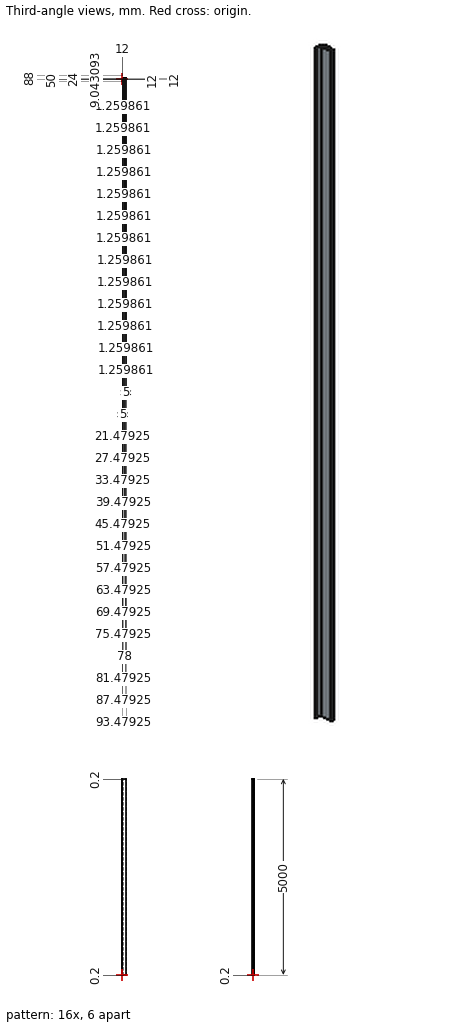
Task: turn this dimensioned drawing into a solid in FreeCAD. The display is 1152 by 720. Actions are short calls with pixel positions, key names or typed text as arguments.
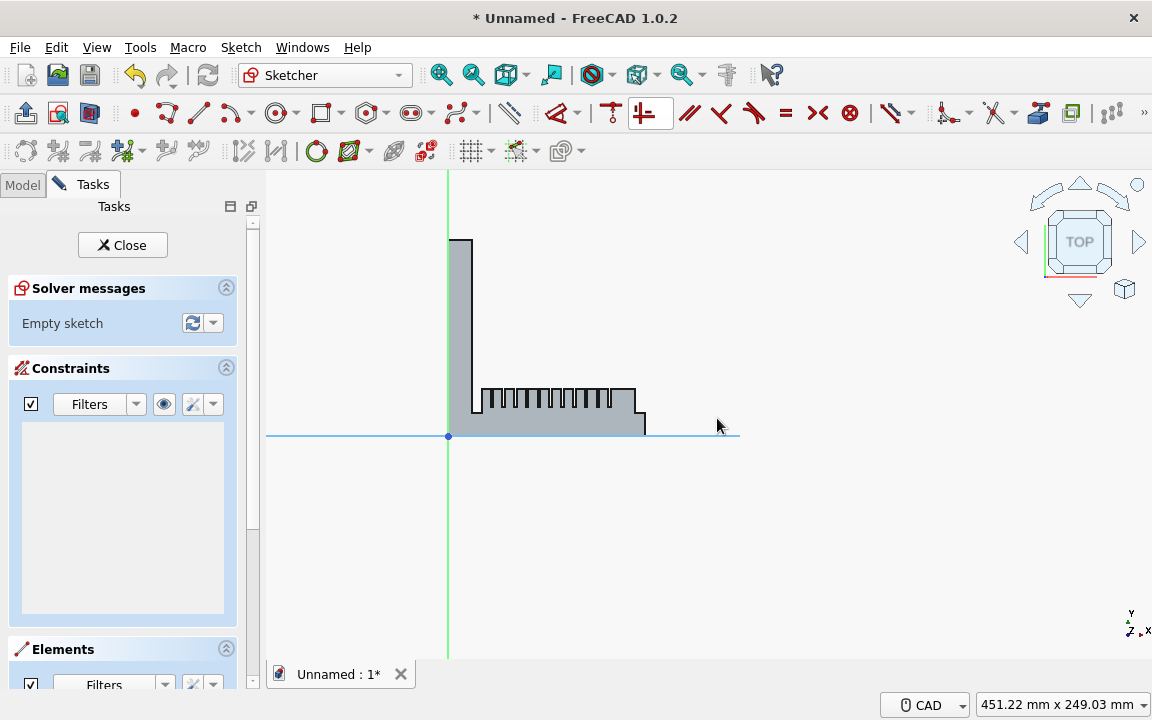
scroll(620, 397, up, 14)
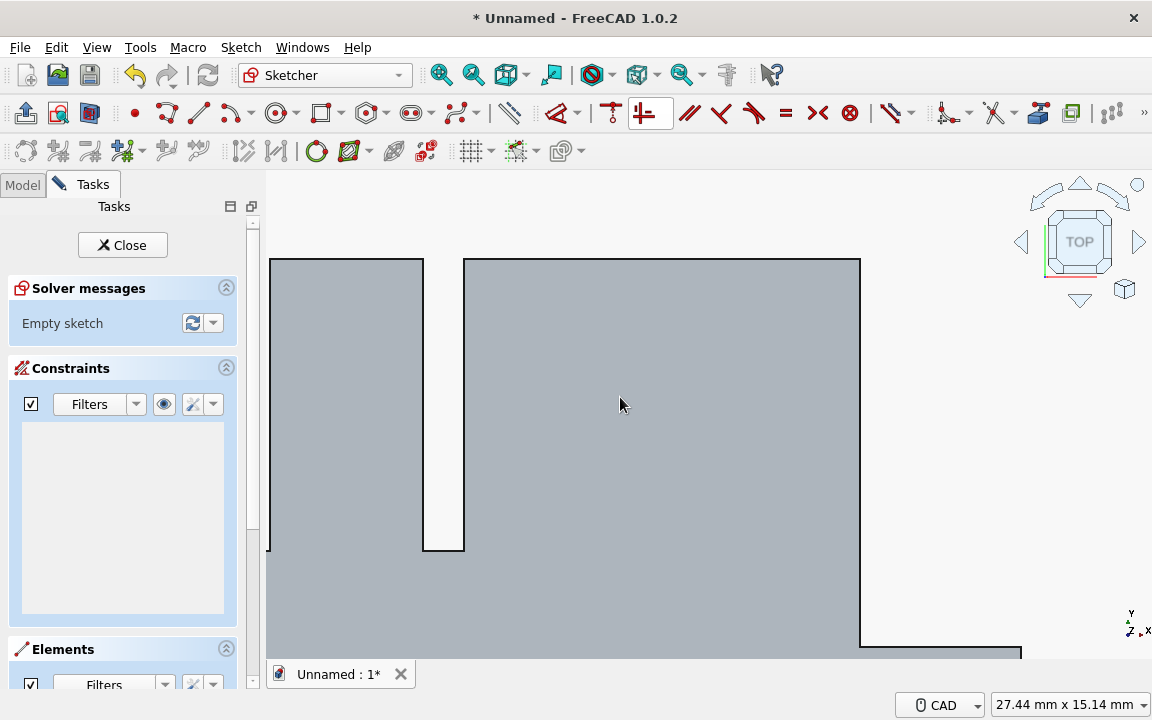
click(322, 114)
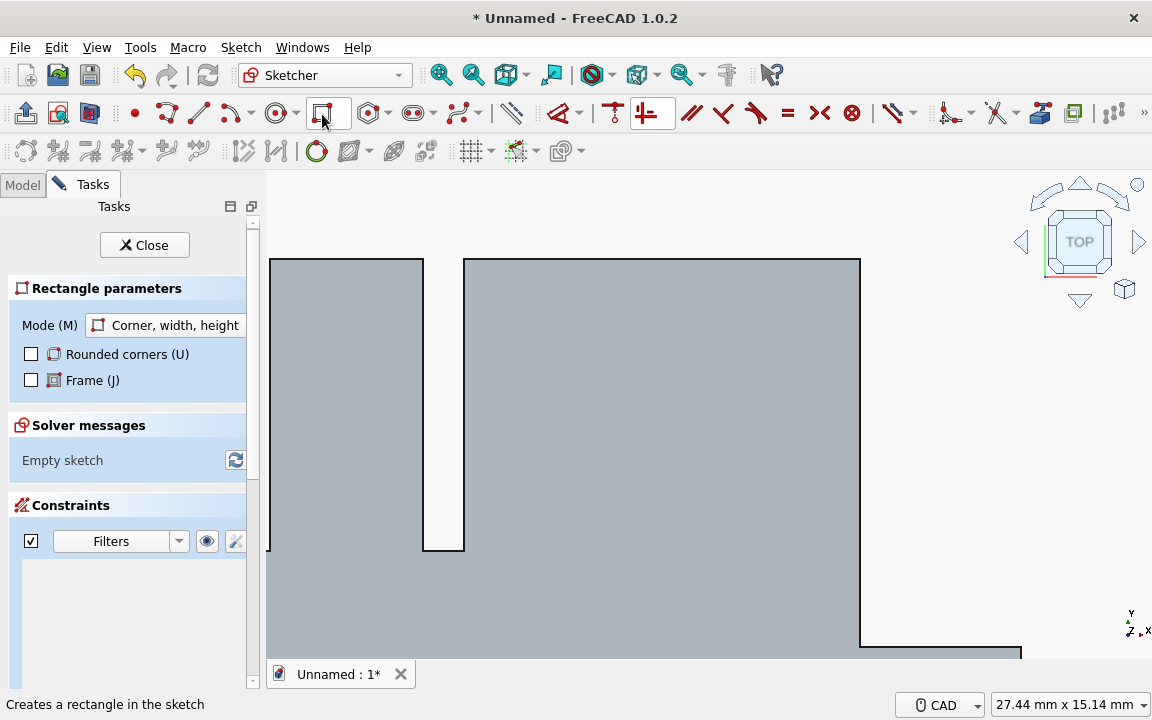
click(617, 259)
click(658, 551)
key(Escape)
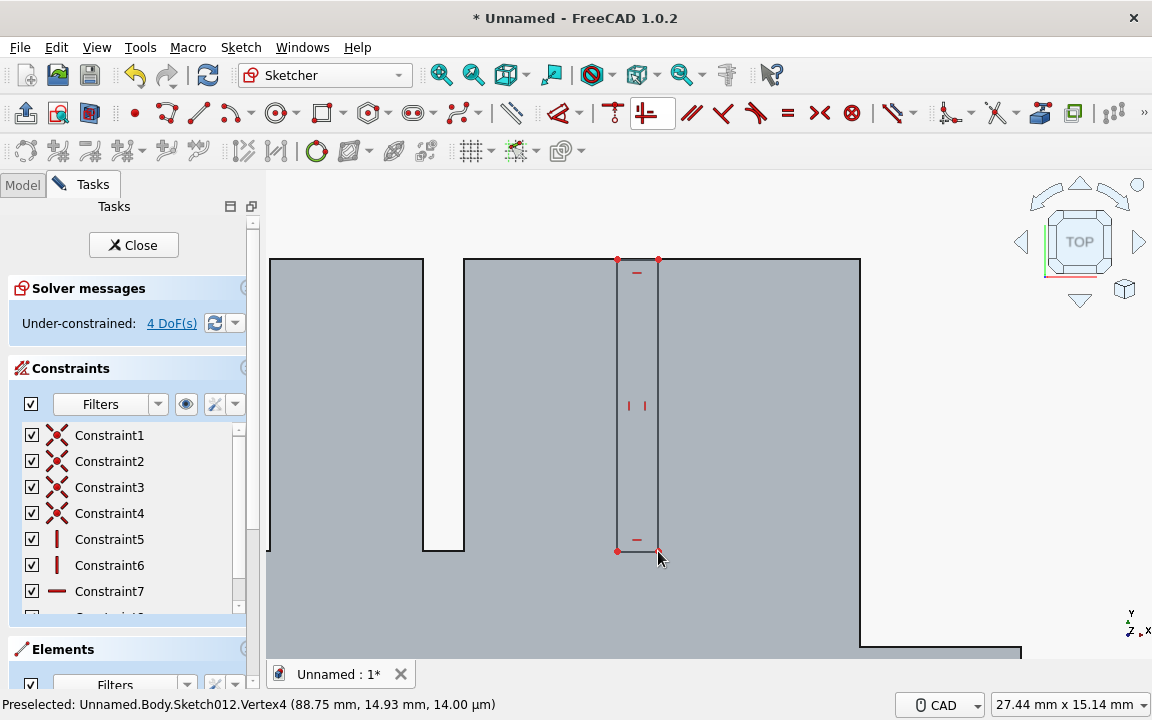
click(558, 114)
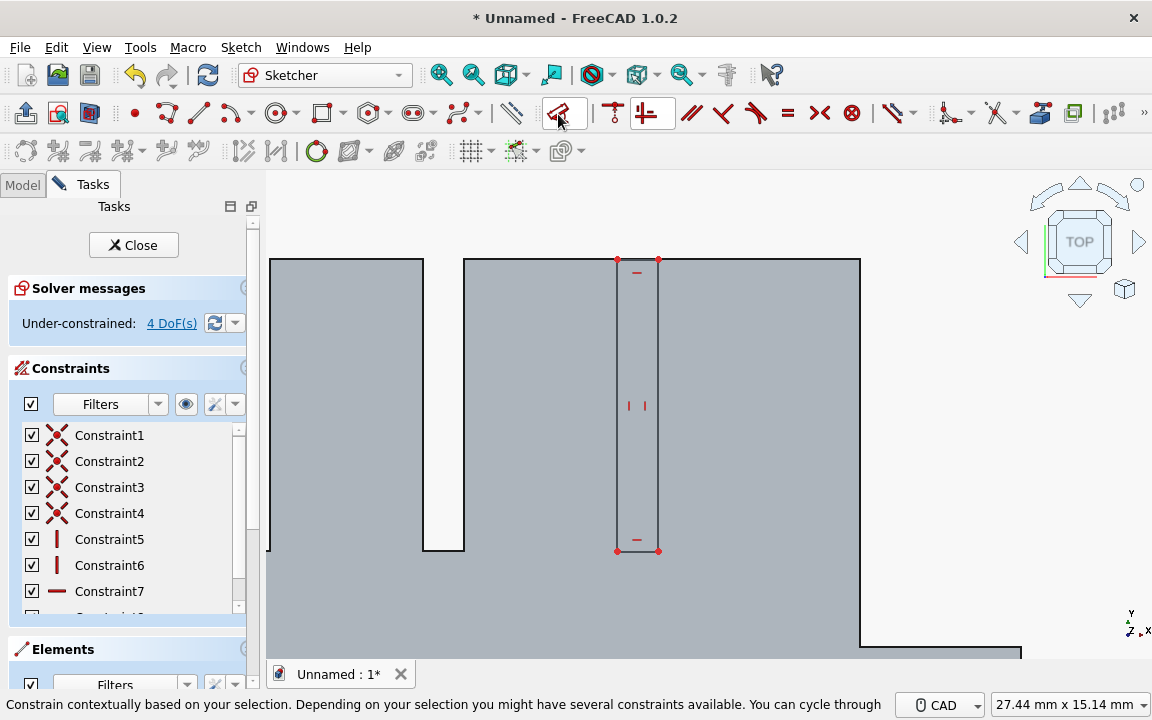
click(617, 260)
click(651, 575)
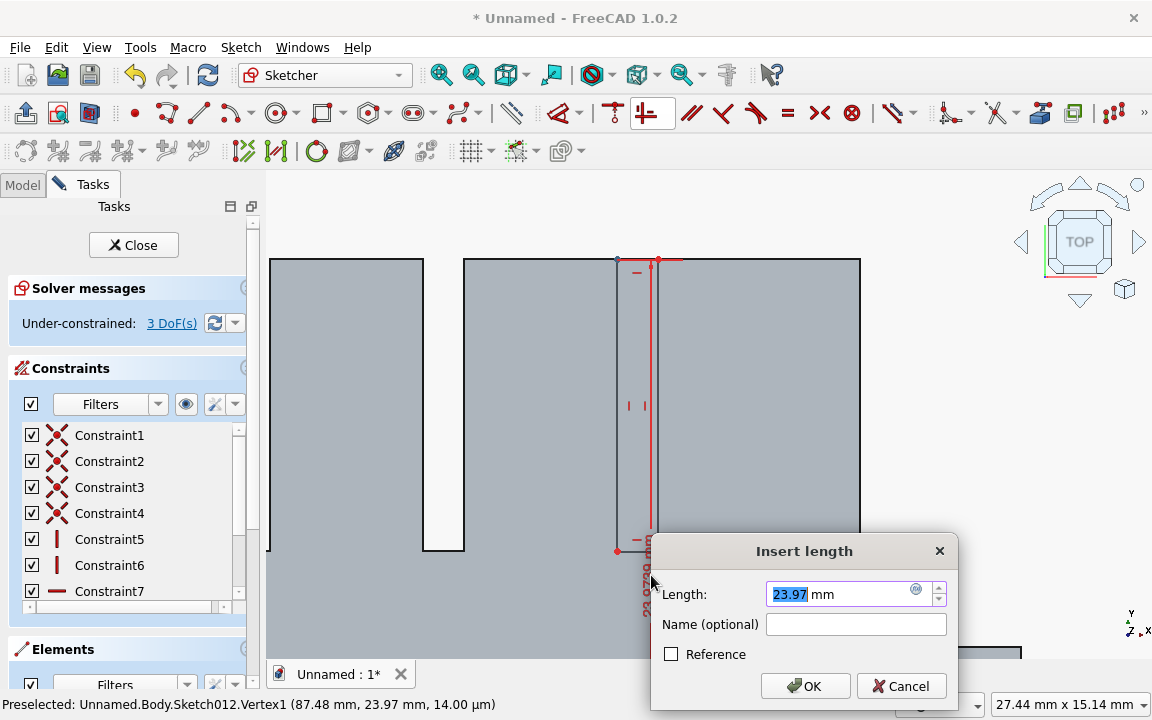
text(24)
key(Return)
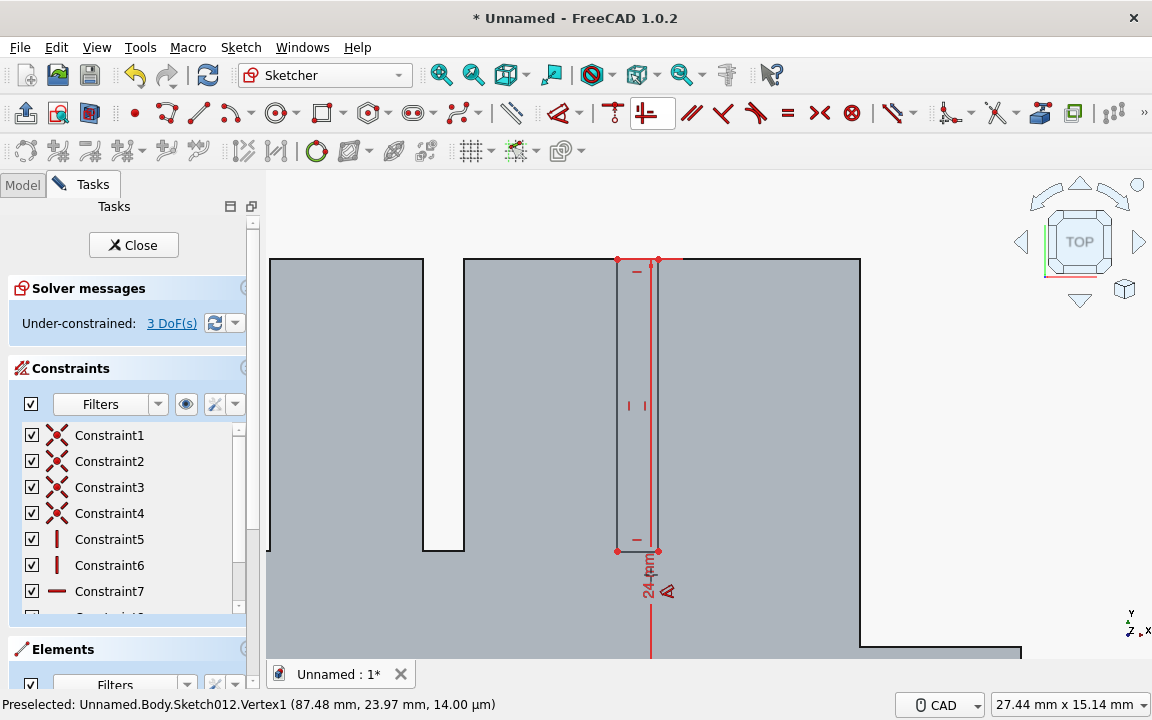
click(617, 347)
click(583, 406)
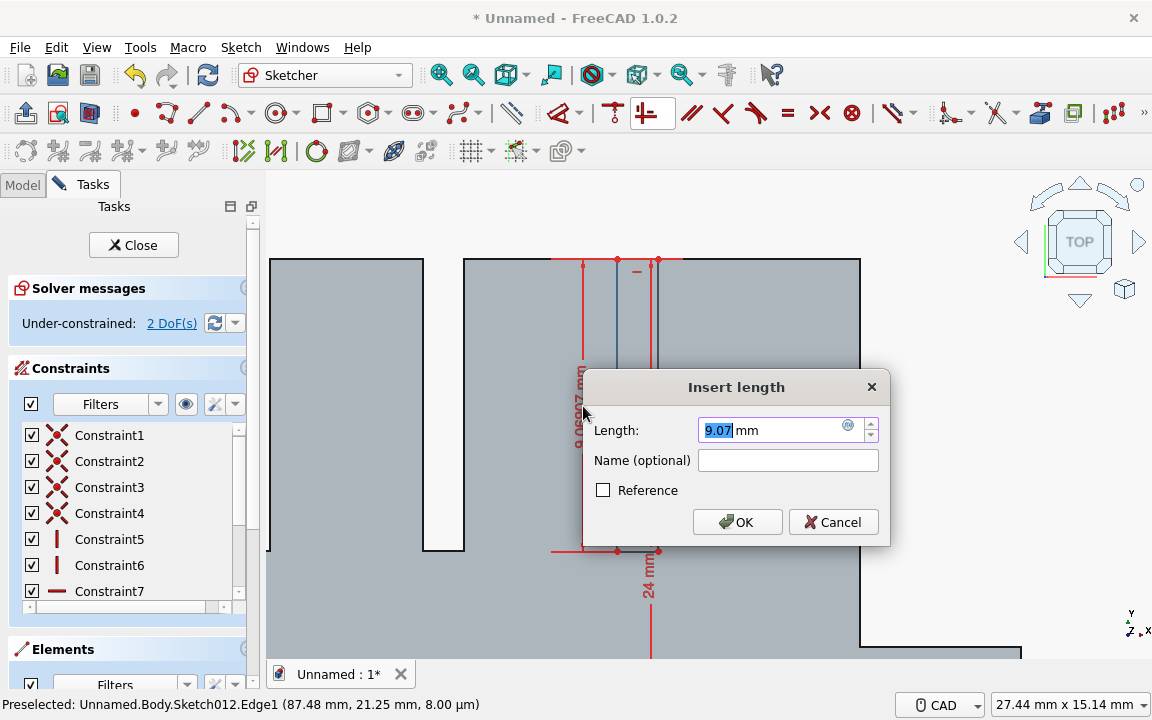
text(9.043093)
key(Return)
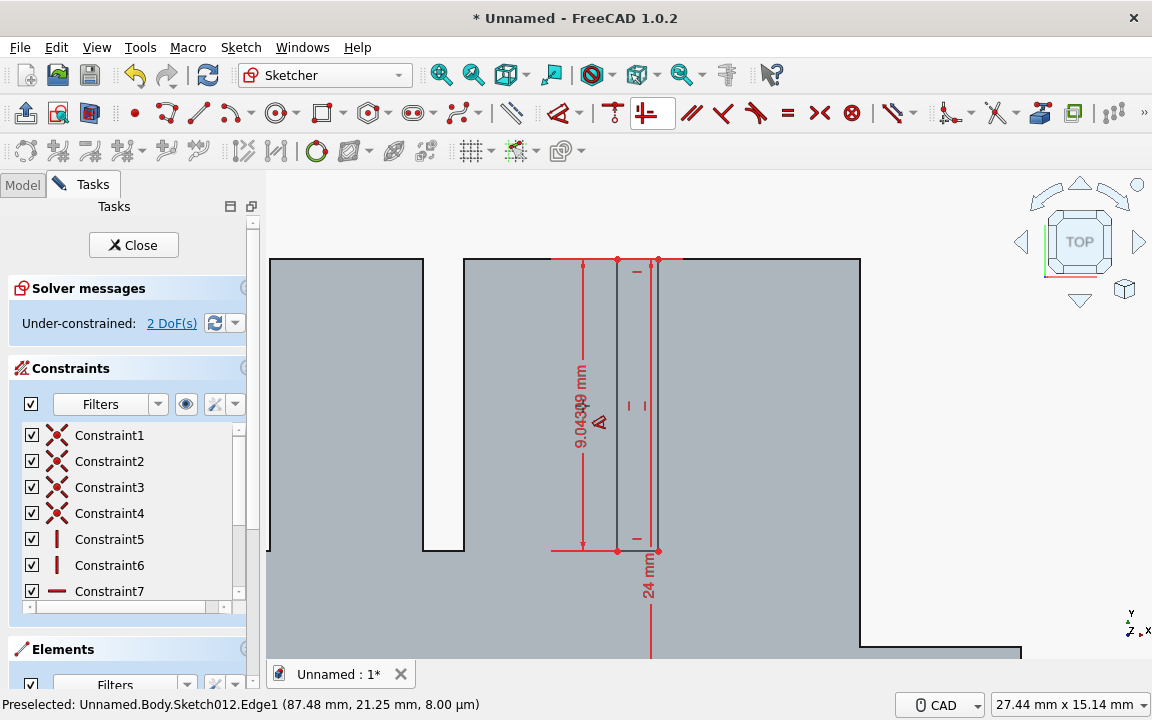
click(629, 551)
click(637, 517)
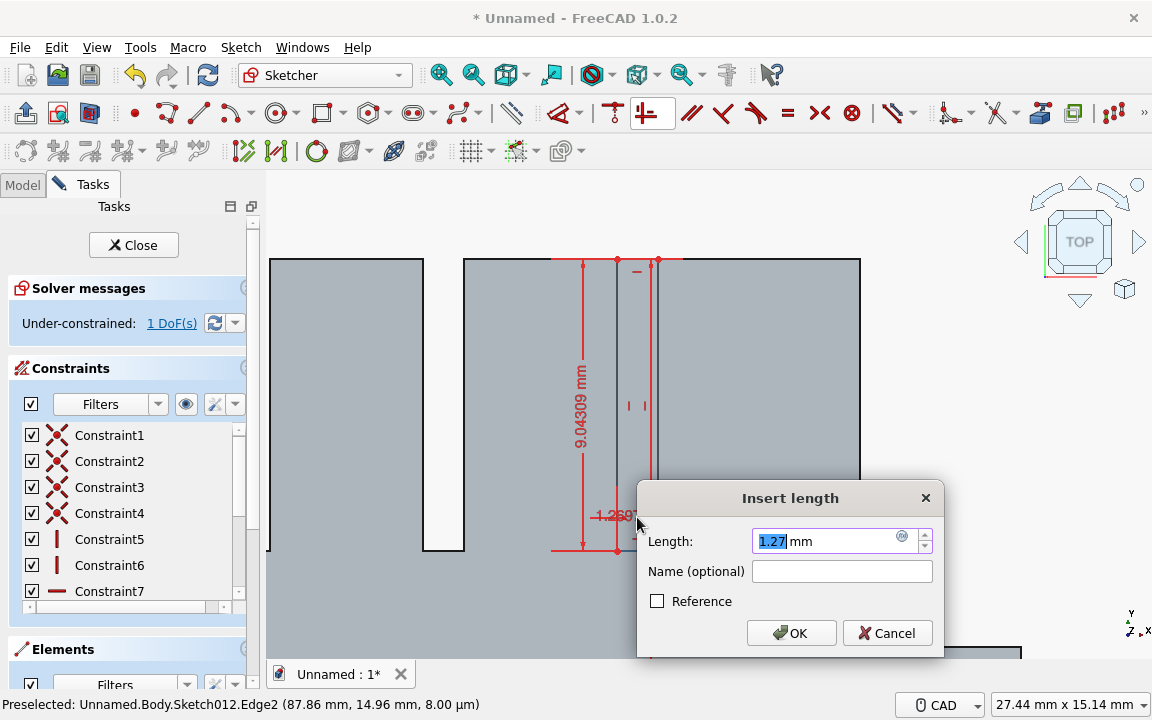
text(1.259861)
key(Return)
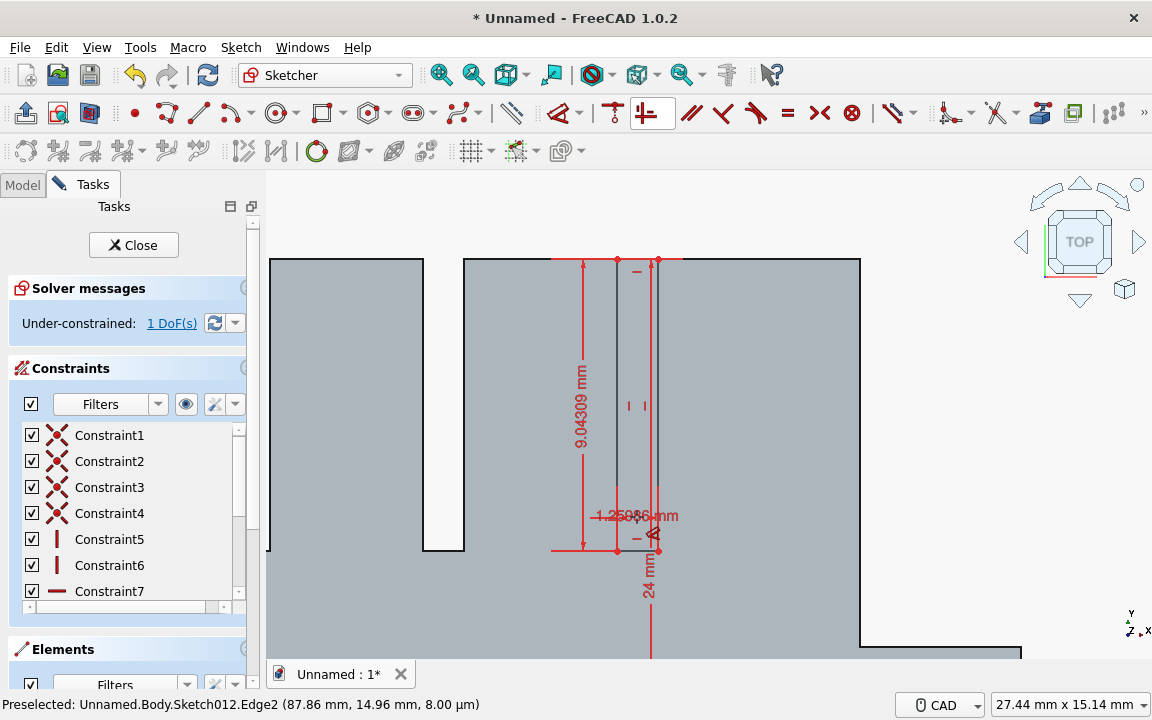
click(617, 259)
click(456, 225)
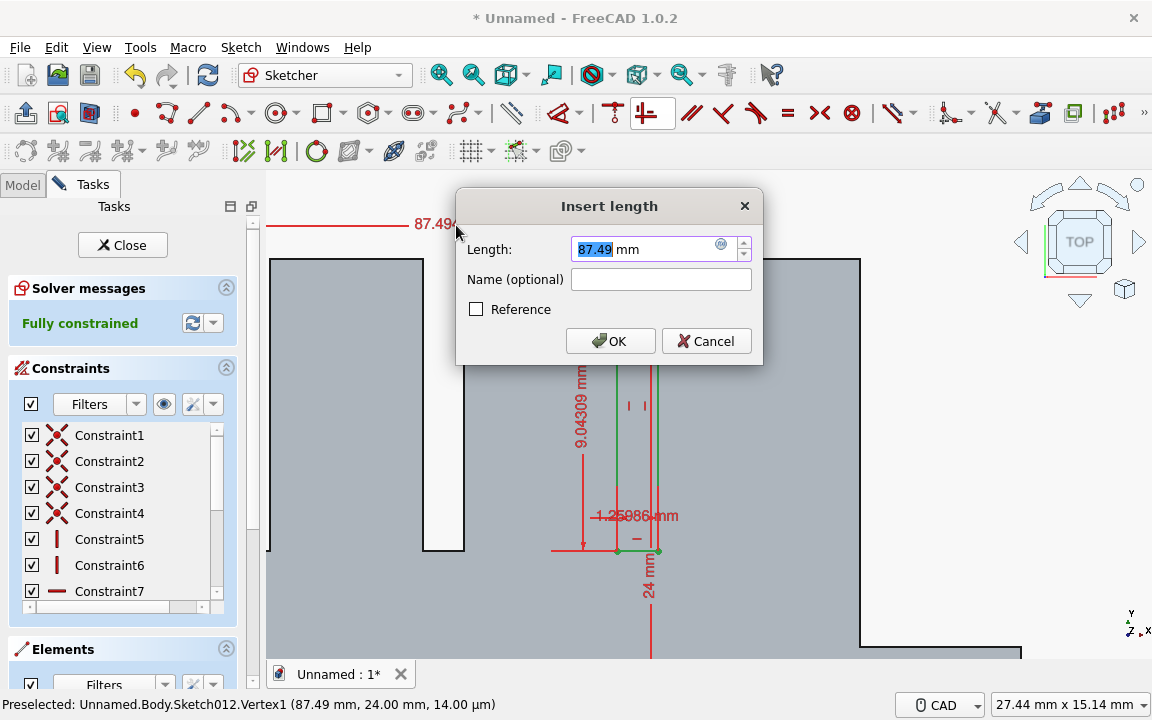
text(87.47925)
key(Return)
key(Escape)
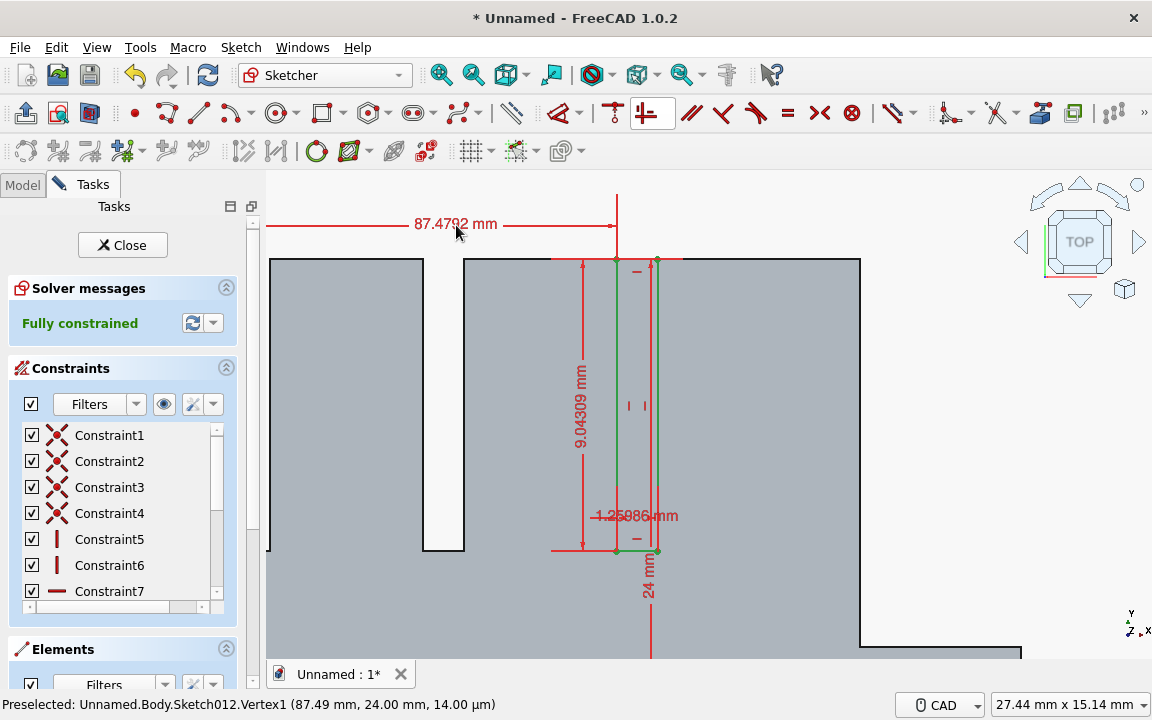
click(123, 245)